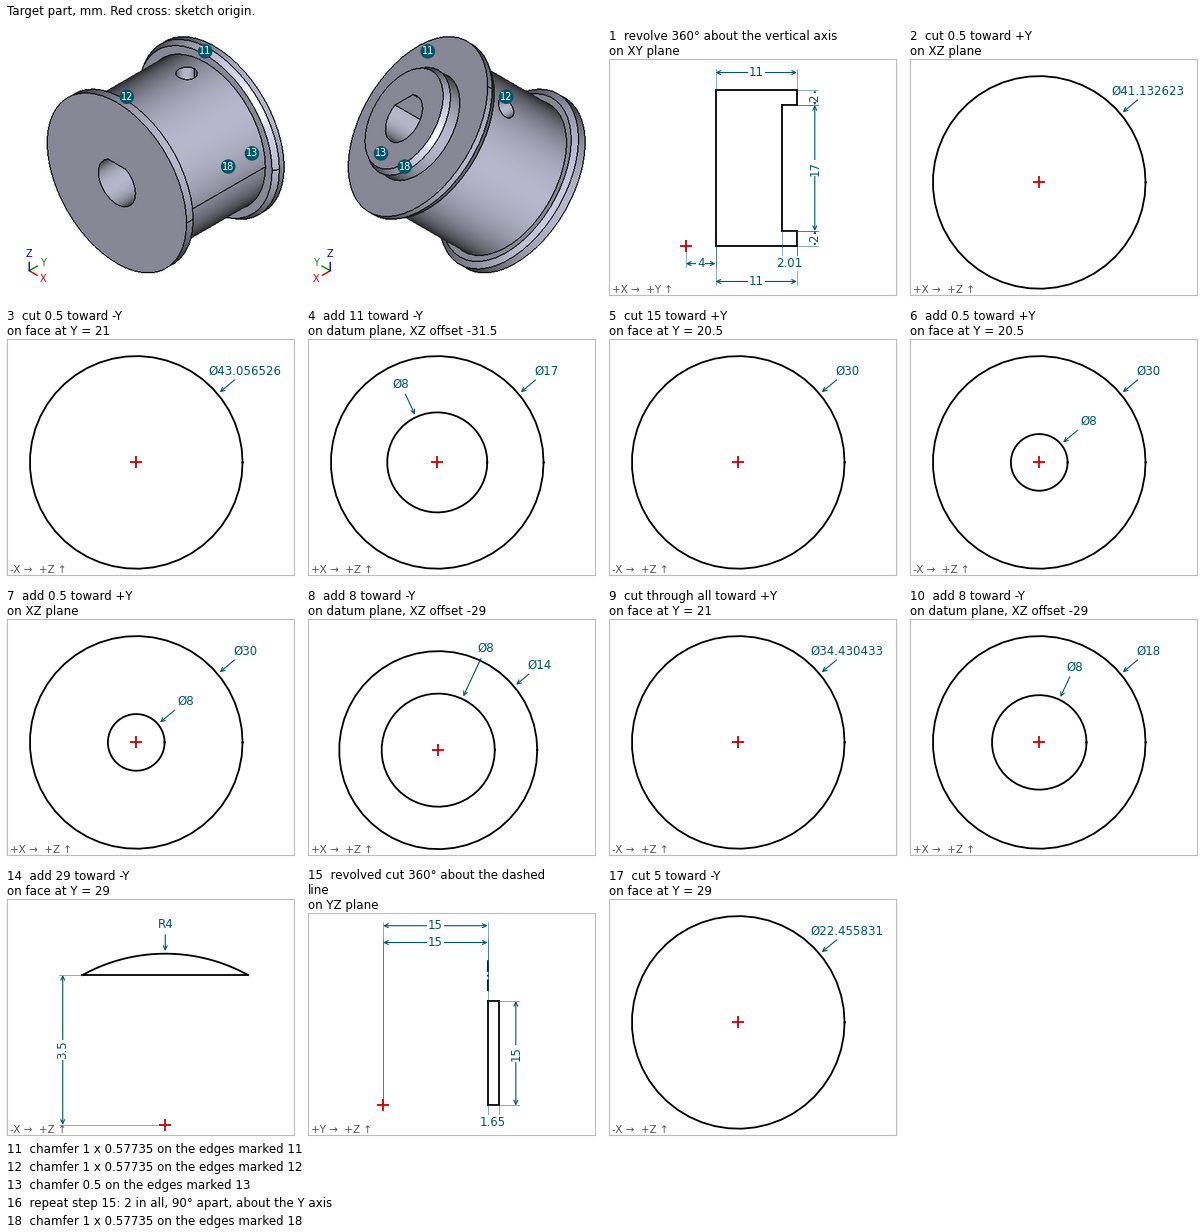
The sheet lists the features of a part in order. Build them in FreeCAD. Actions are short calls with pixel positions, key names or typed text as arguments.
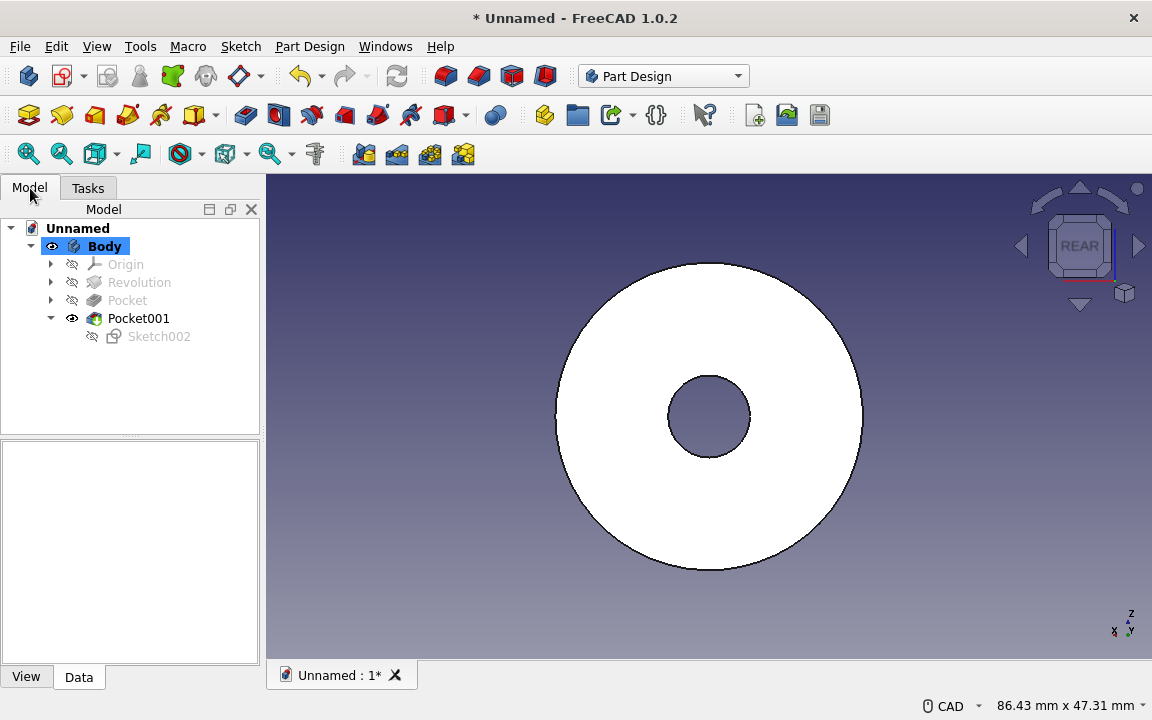
click(51, 264)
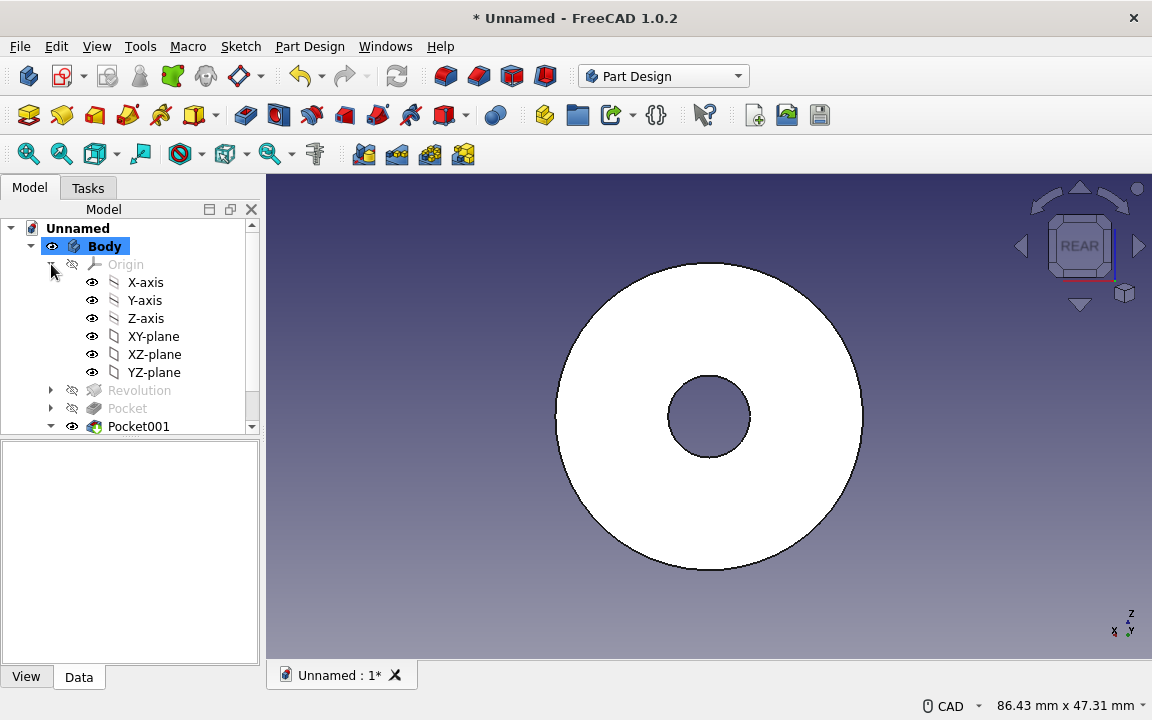
click(137, 354)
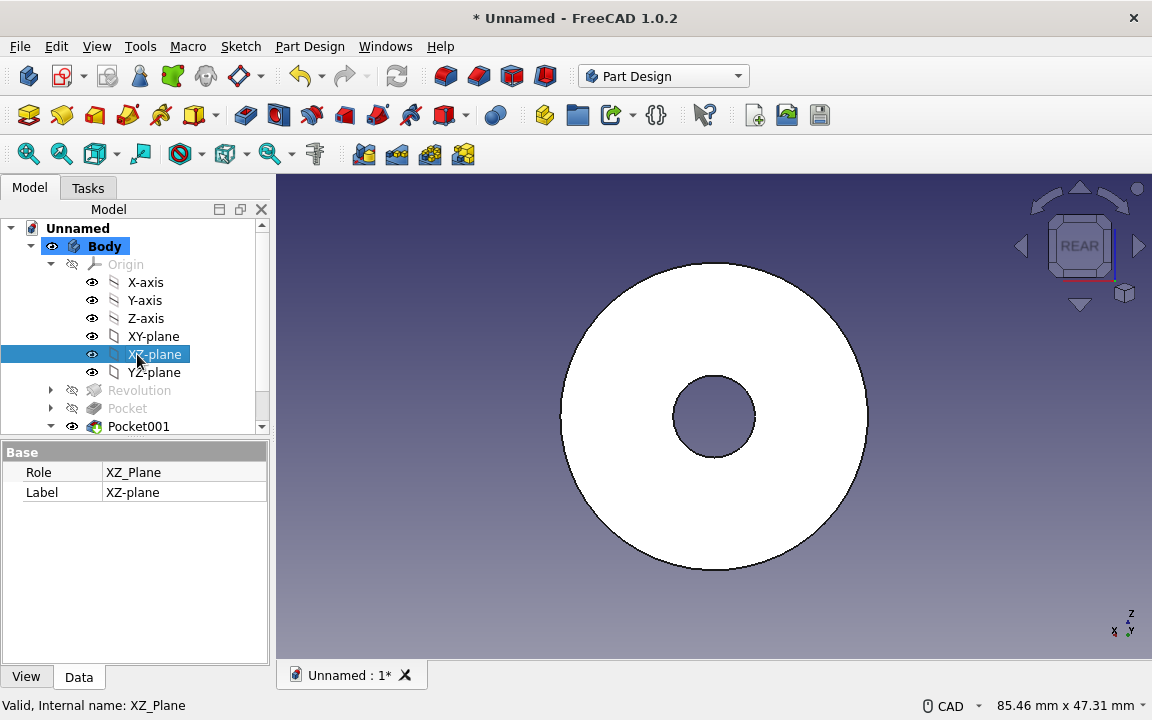
click(238, 76)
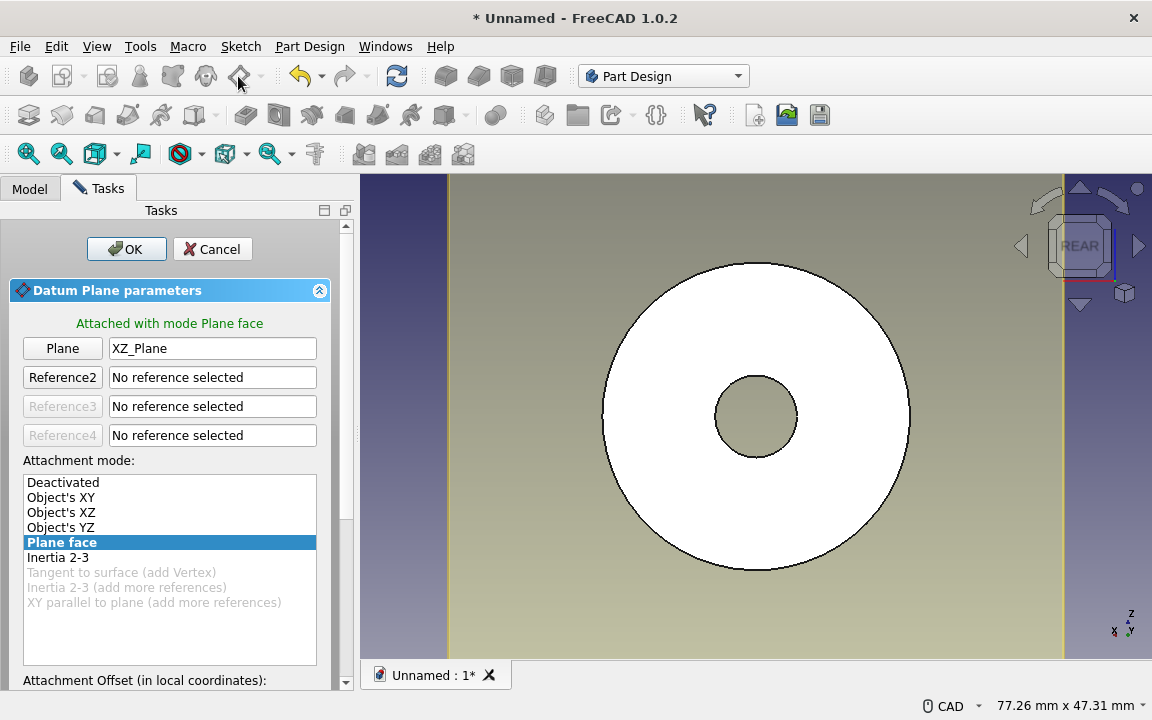
scroll(346, 455, down, 3)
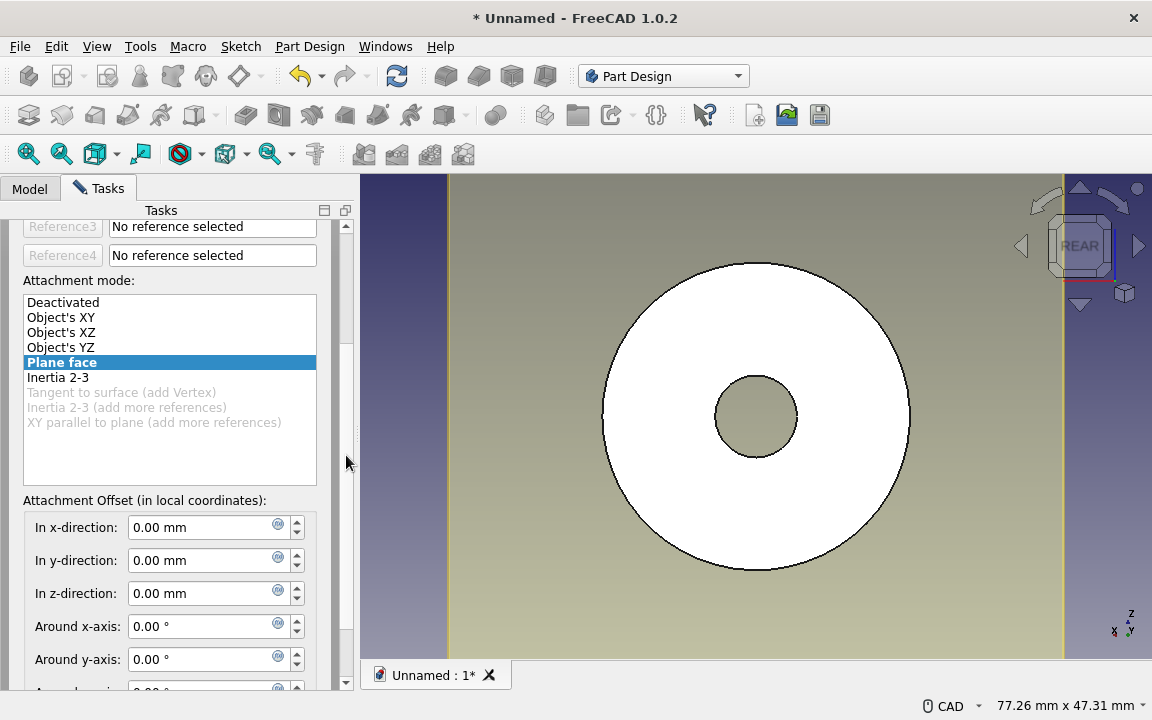
triple_click(210, 594)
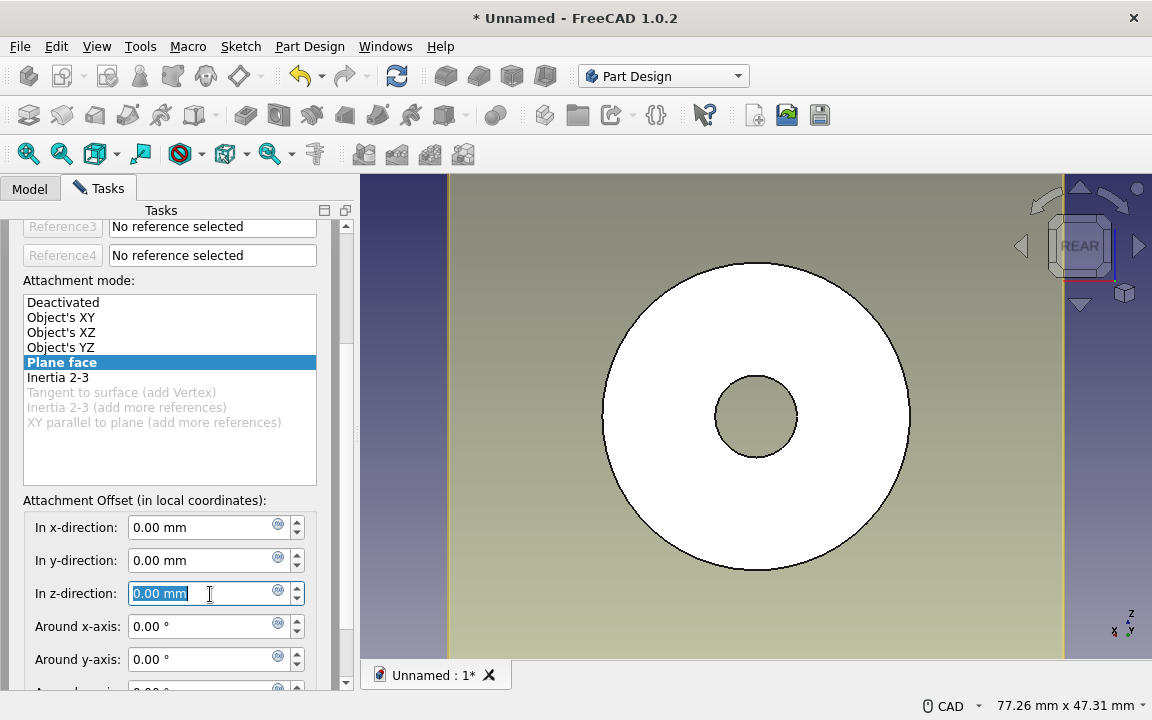
text(-31.5)
key(Tab)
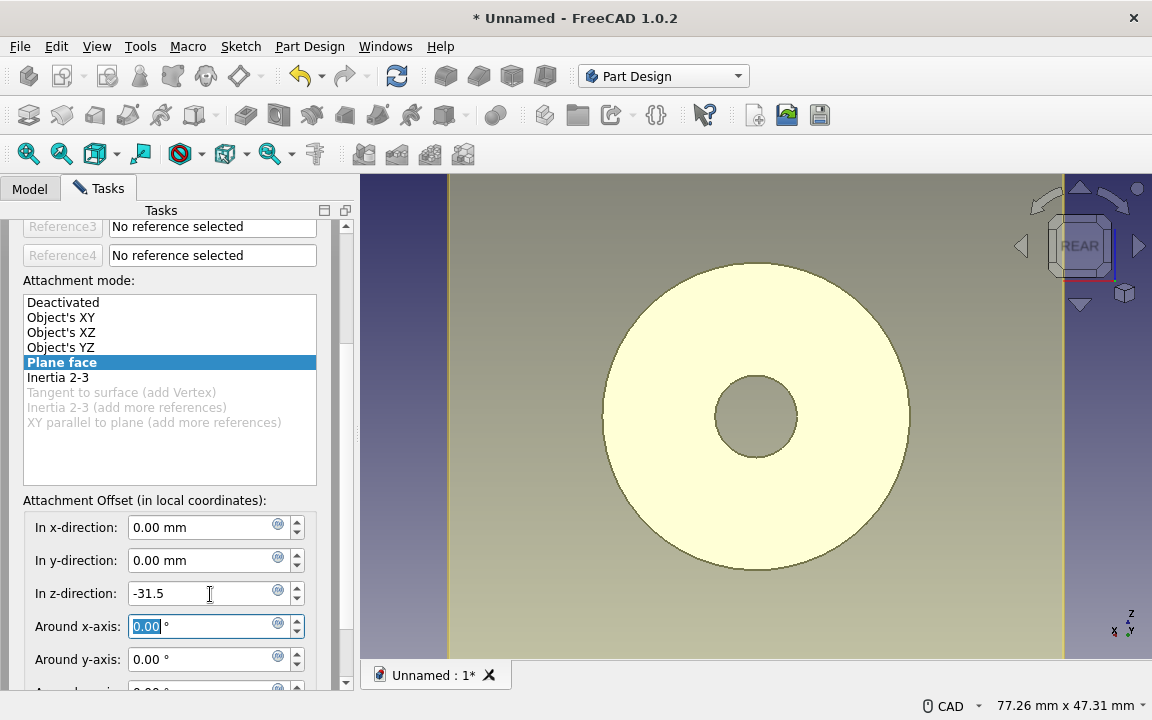
scroll(346, 455, up, 4)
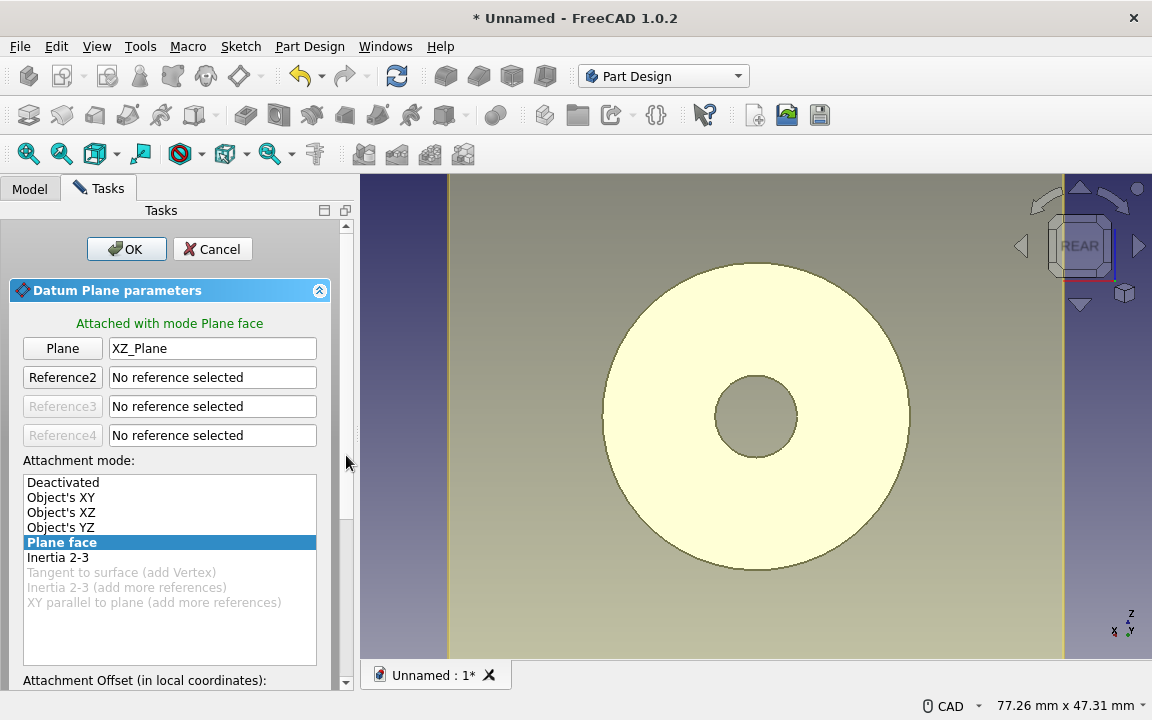
click(127, 249)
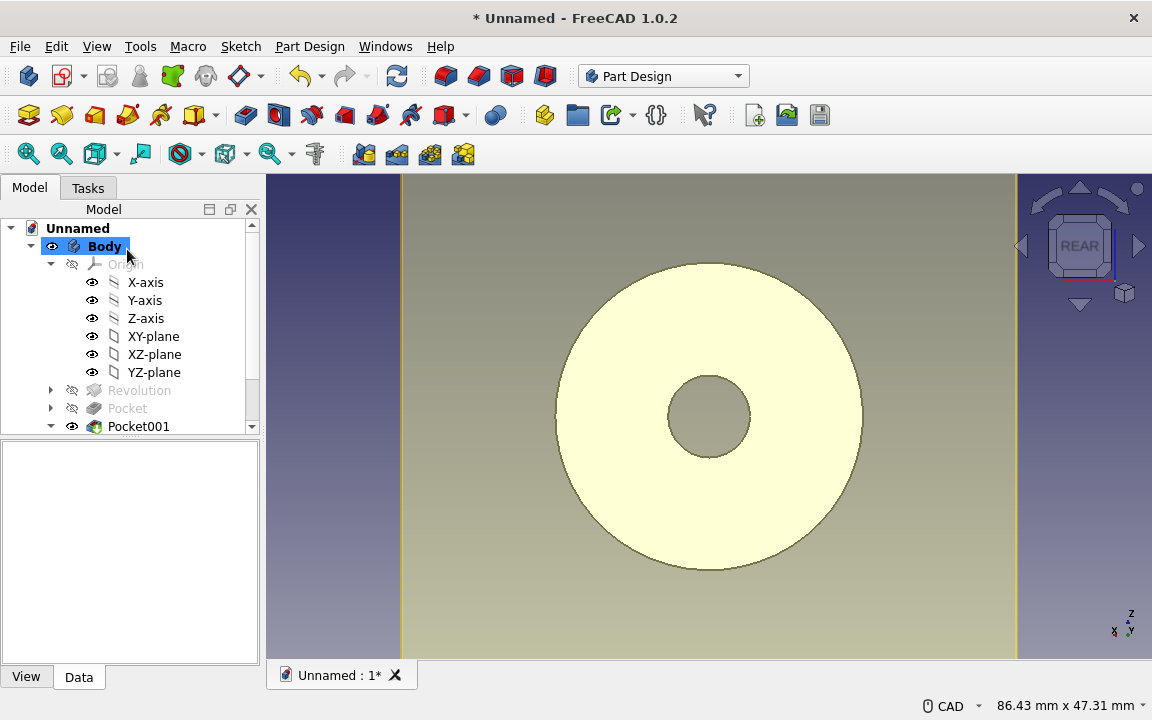
scroll(101, 332, down, 3)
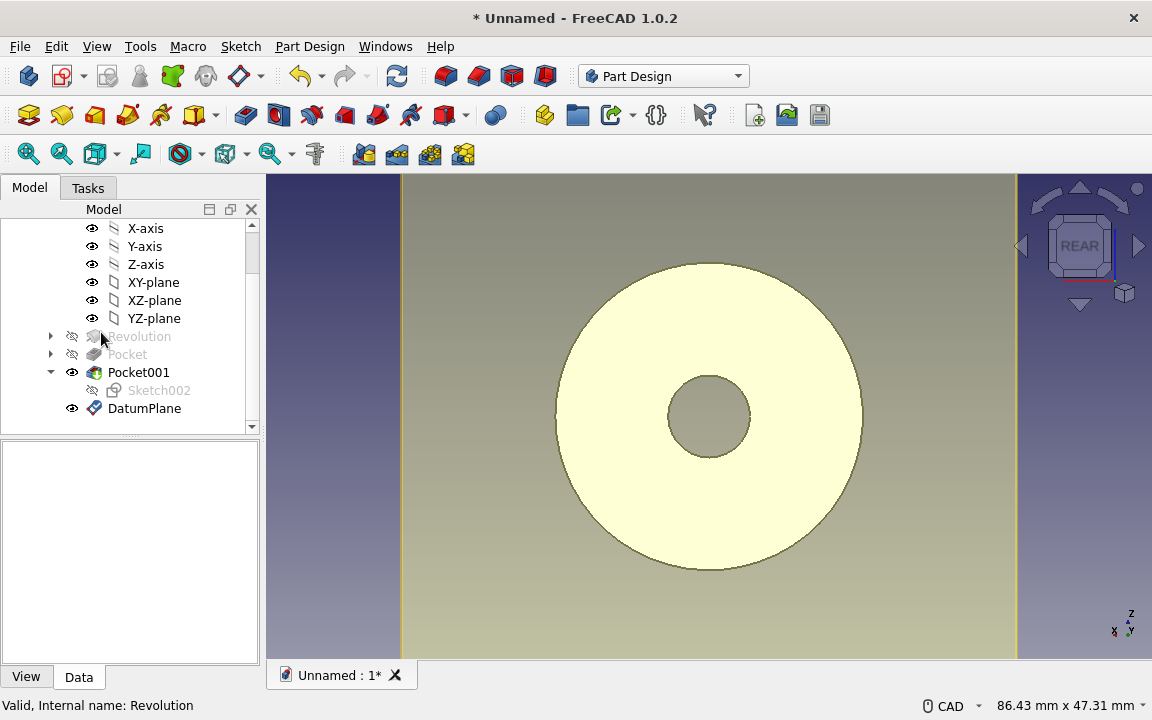
click(117, 408)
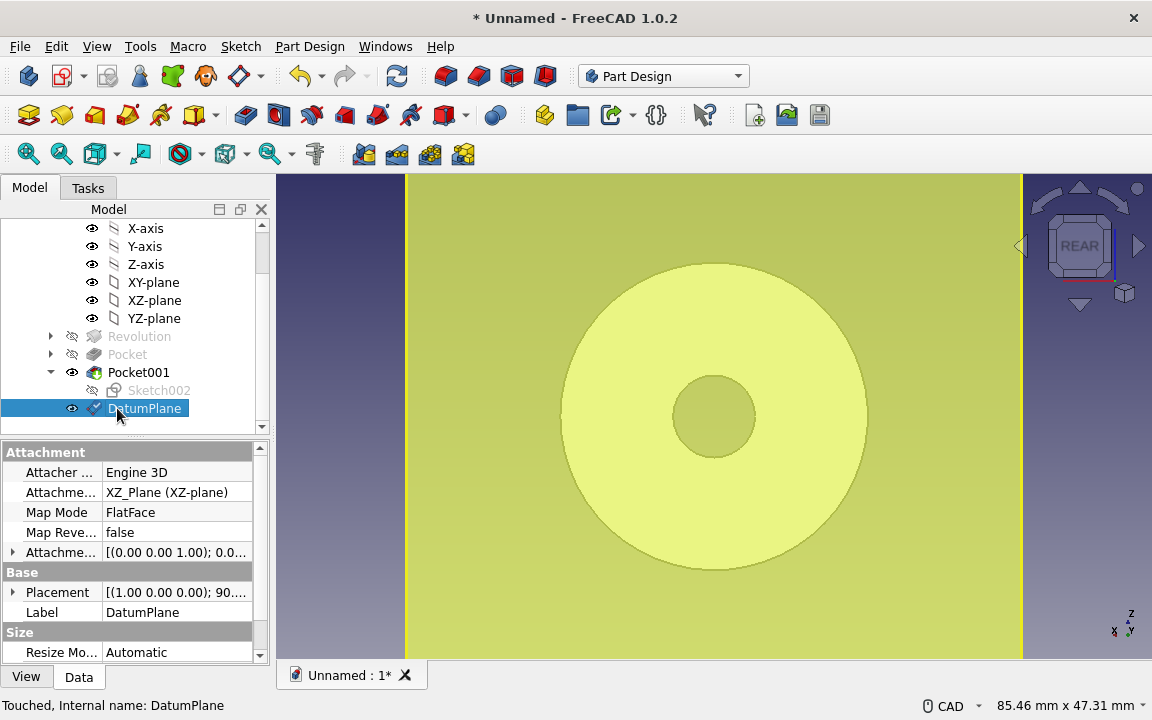
click(62, 76)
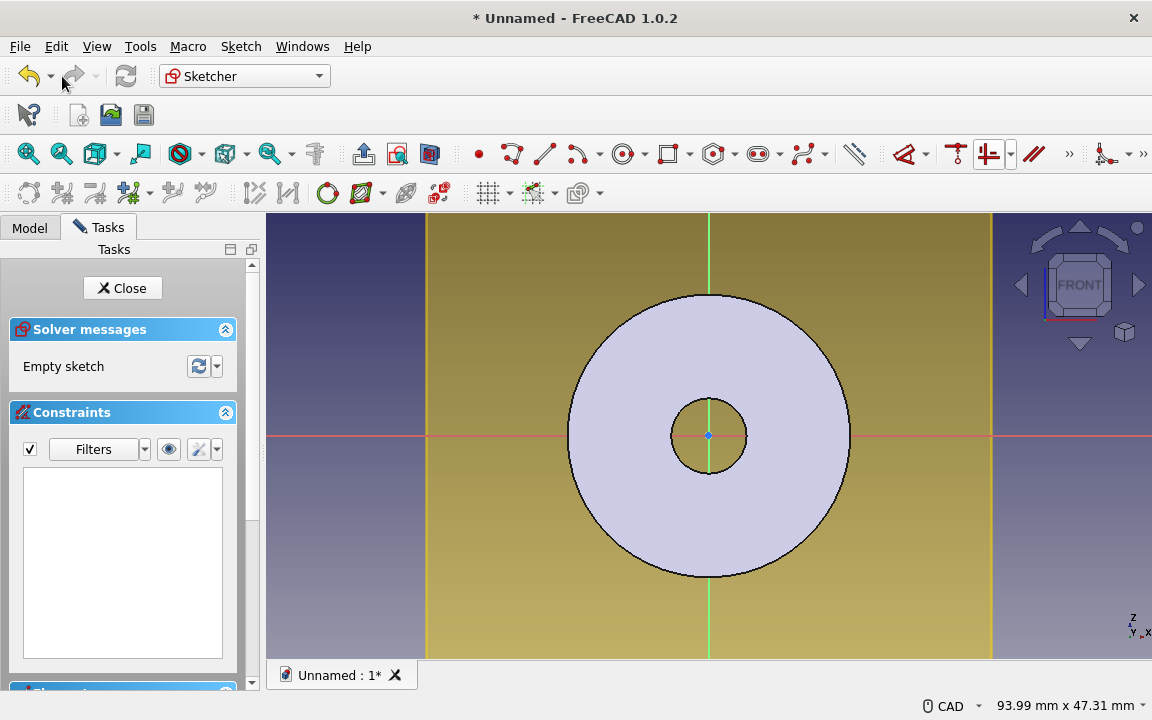
click(430, 154)